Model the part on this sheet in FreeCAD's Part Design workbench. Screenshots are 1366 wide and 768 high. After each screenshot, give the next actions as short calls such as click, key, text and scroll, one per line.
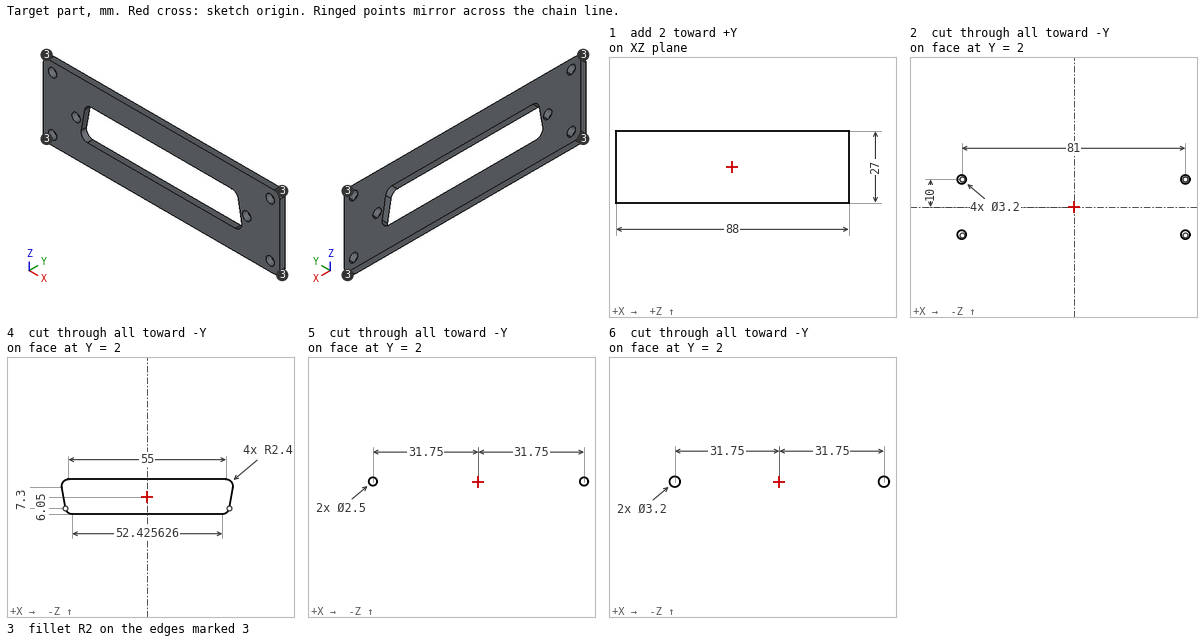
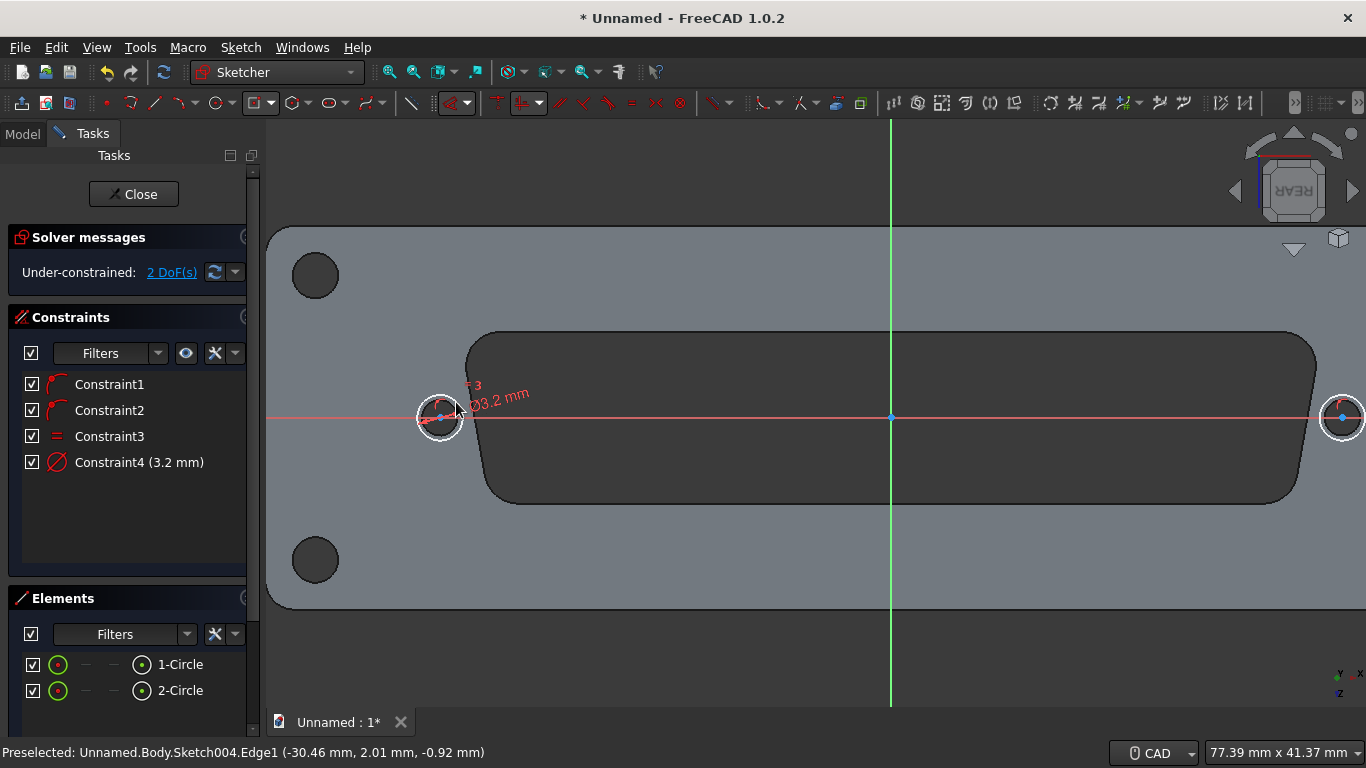
click(440, 418)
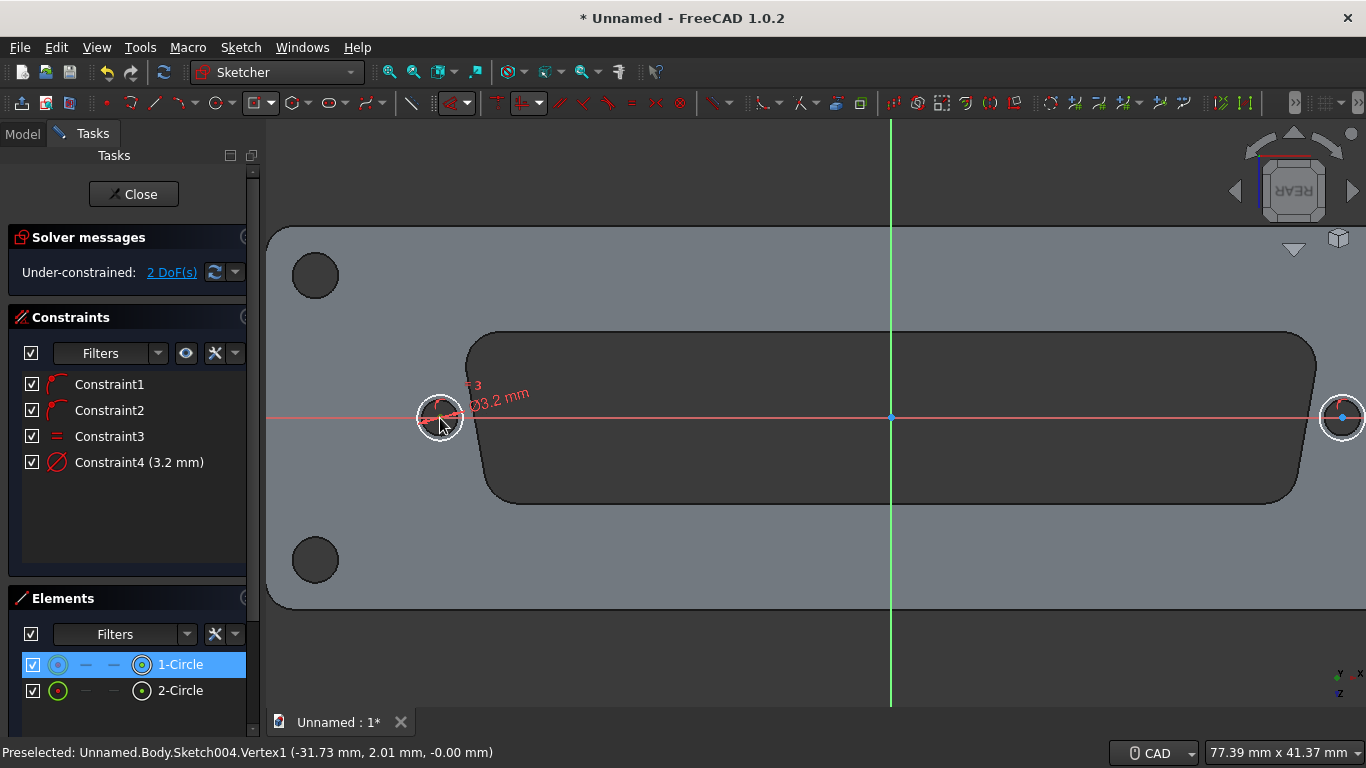
key(l)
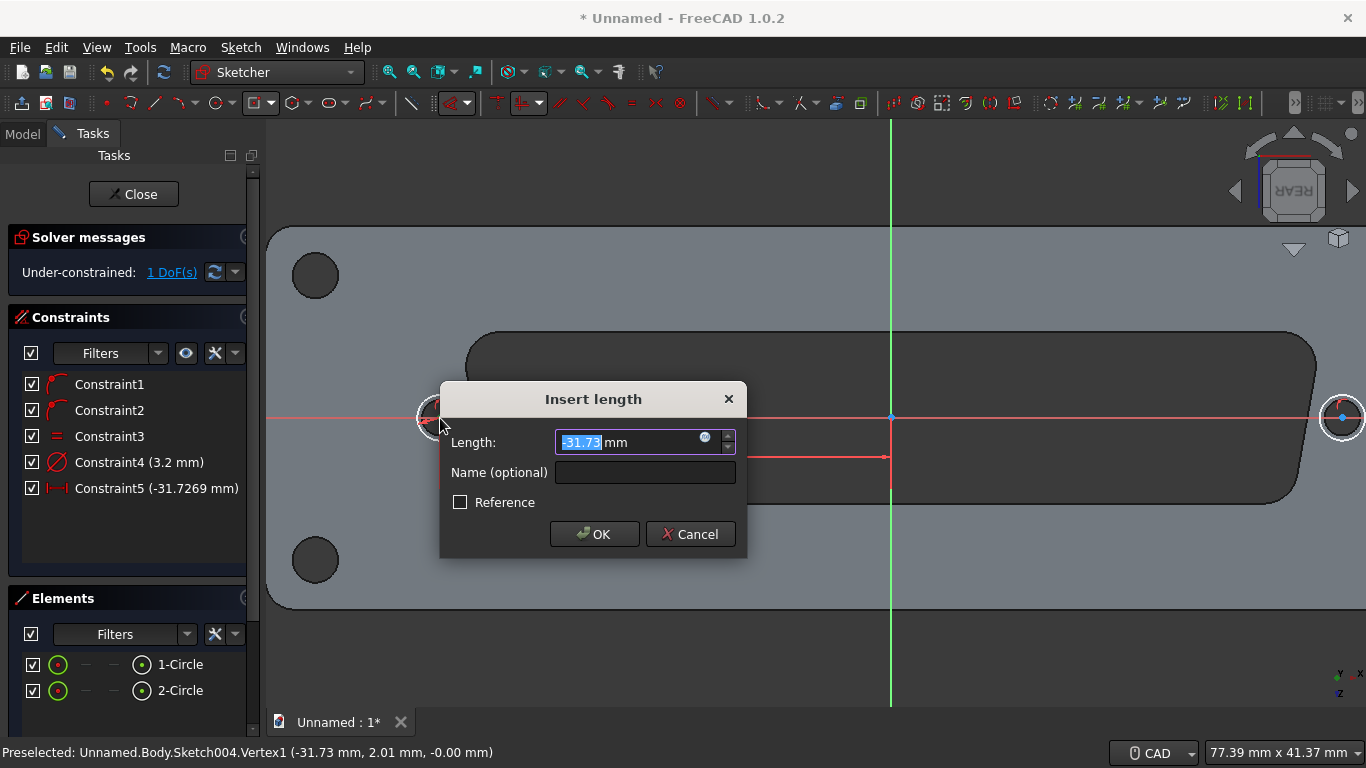
text(-31.75)
key(Return)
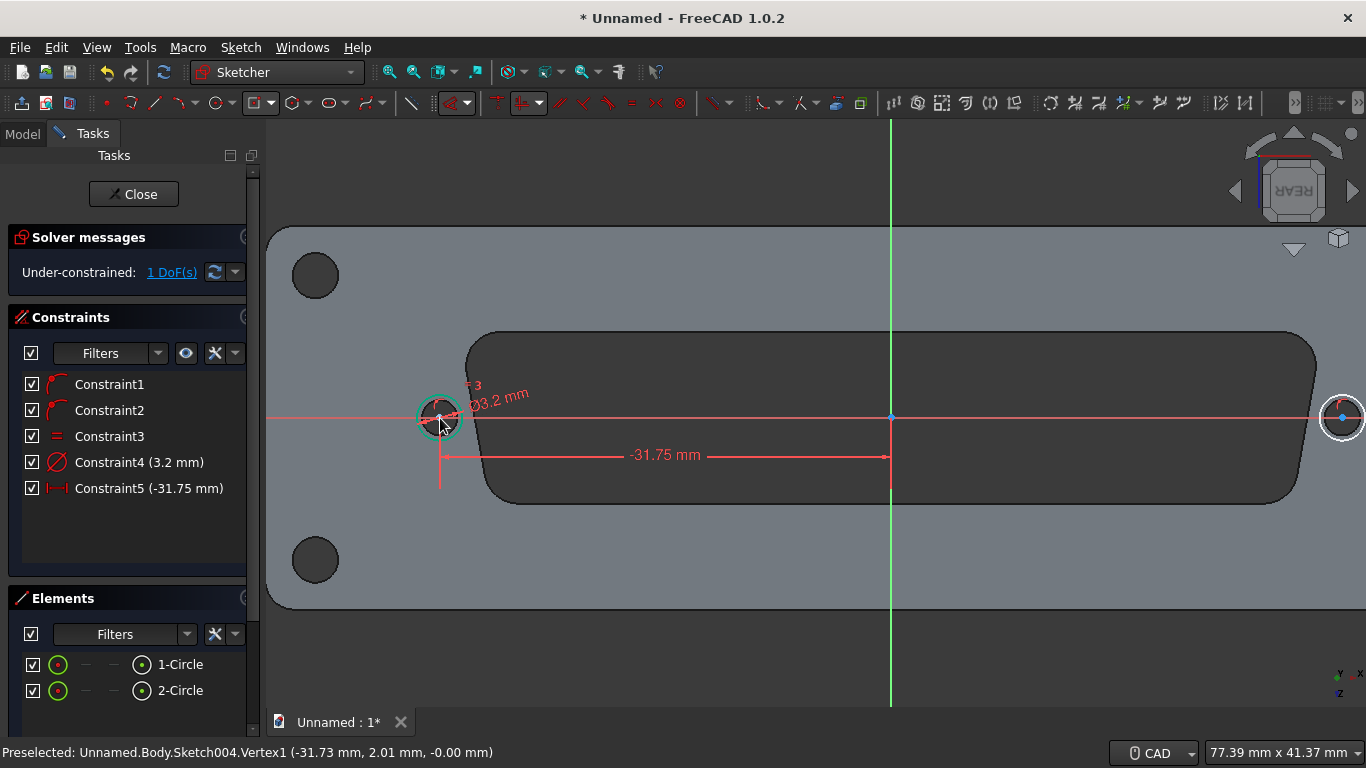
scroll(456, 403, down, 2)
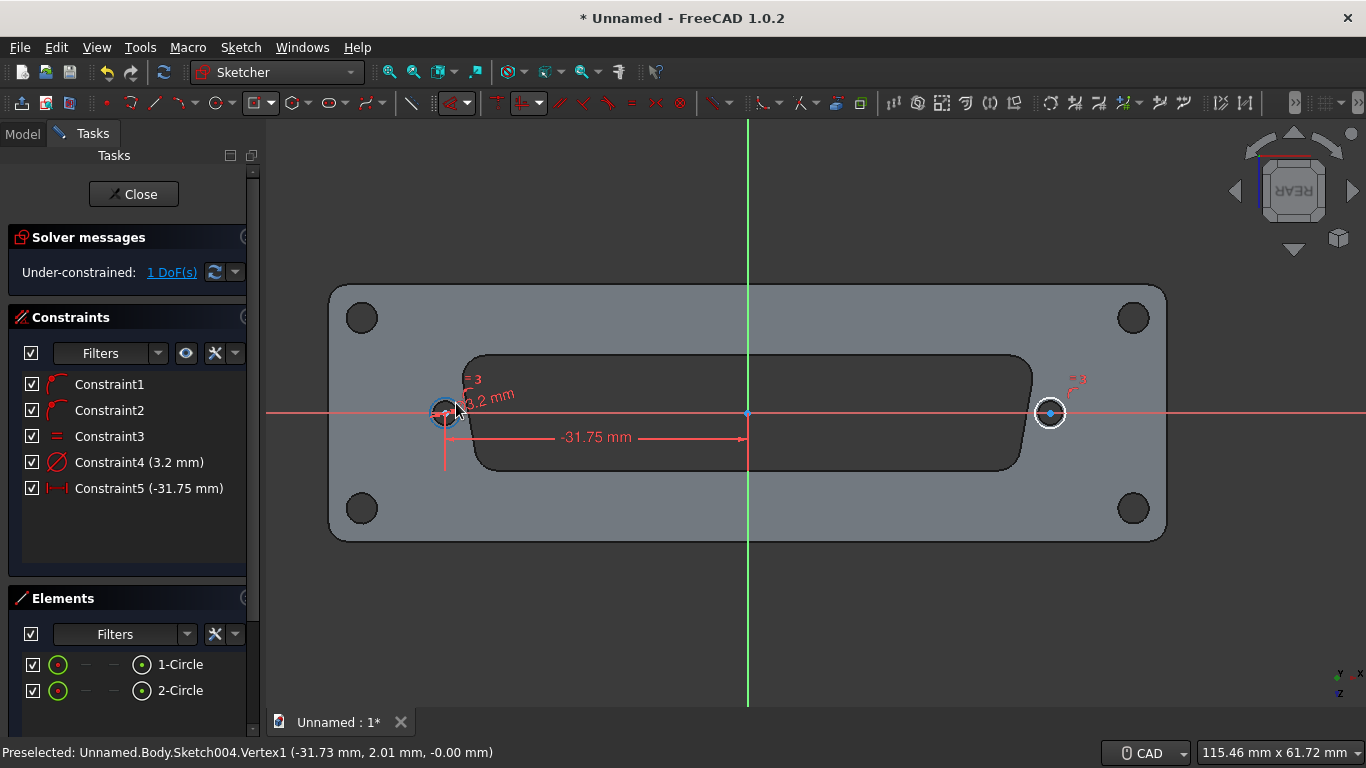
click(1050, 413)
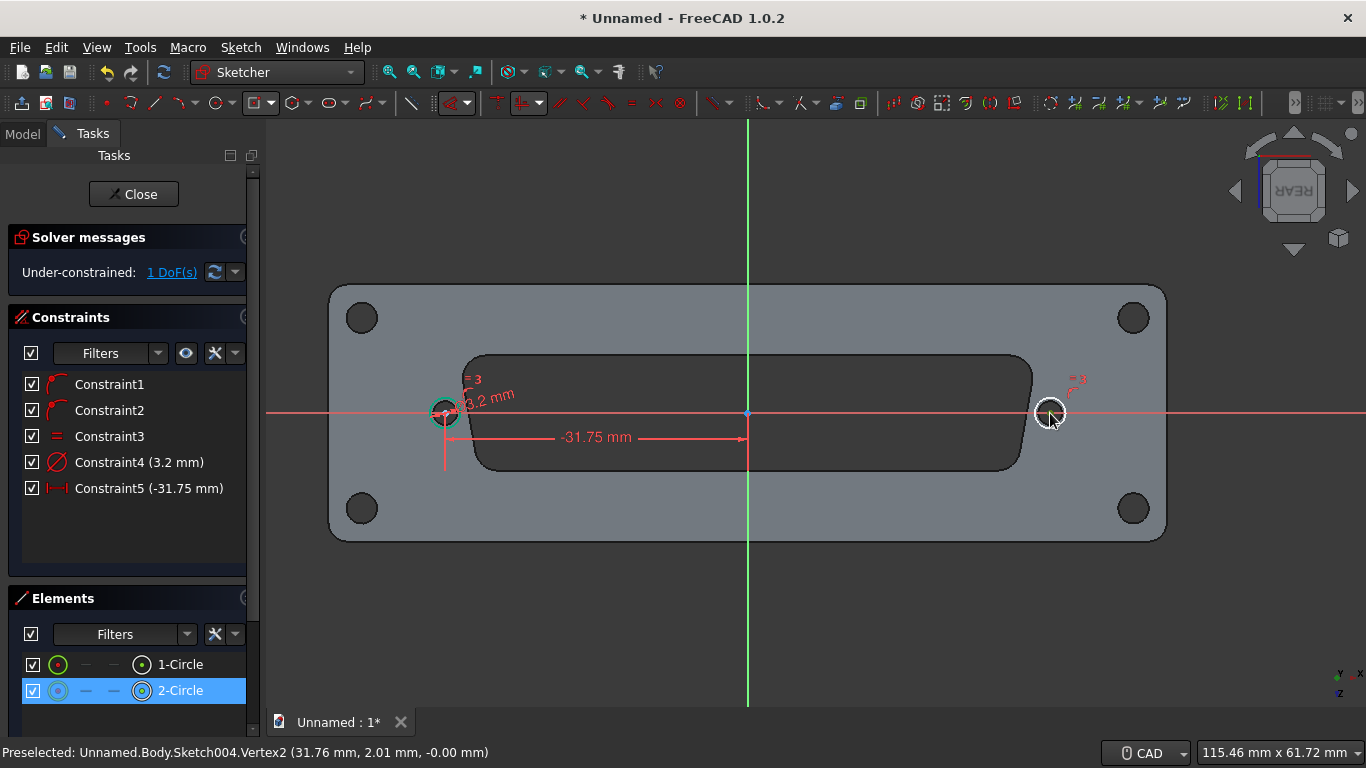
click(470, 104)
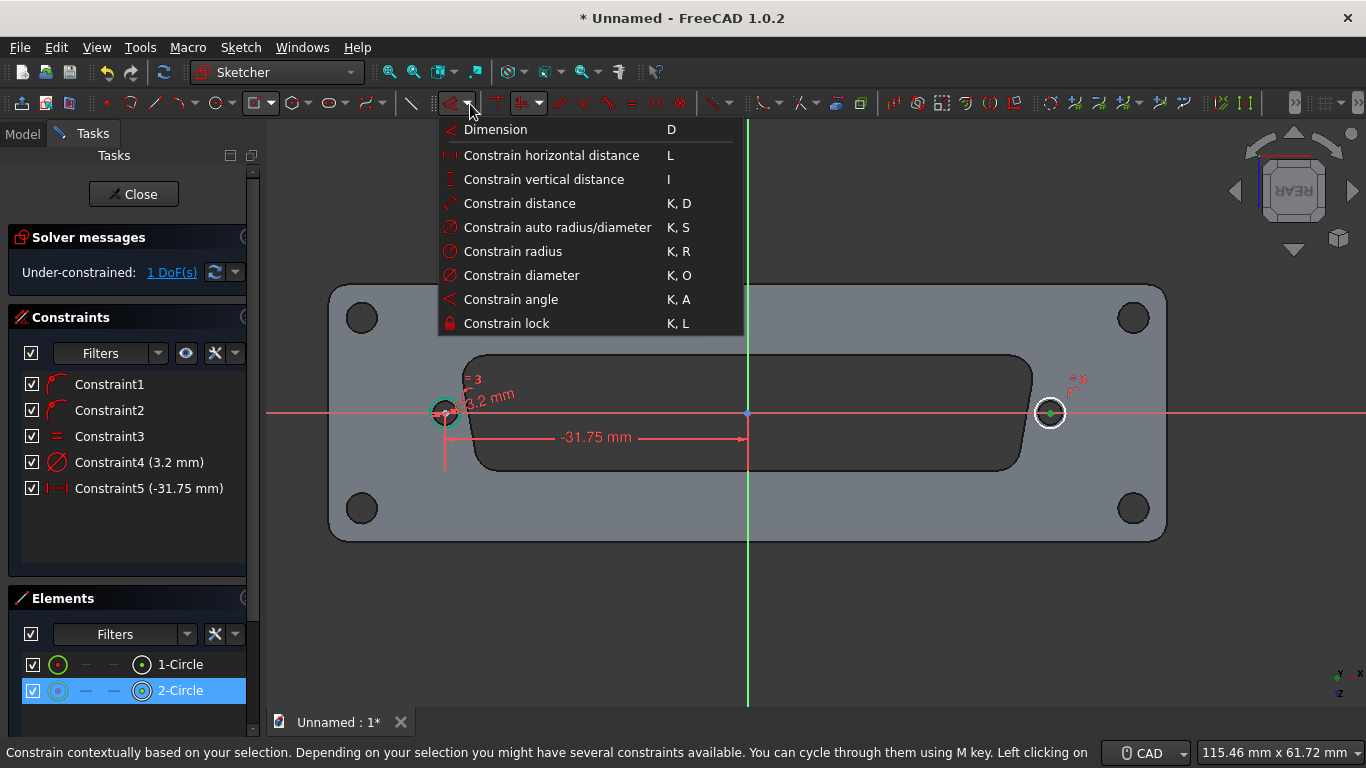
click(591, 155)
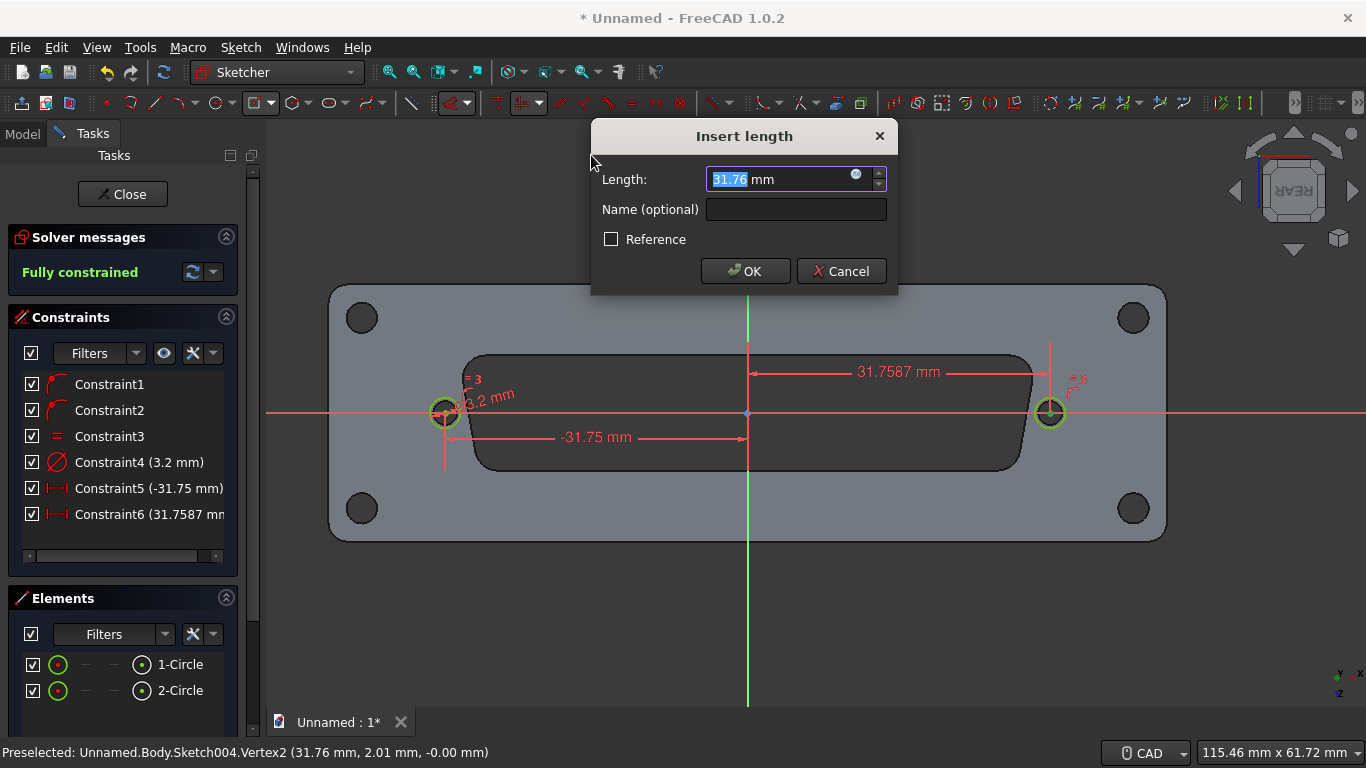
text(31.75)
key(Return)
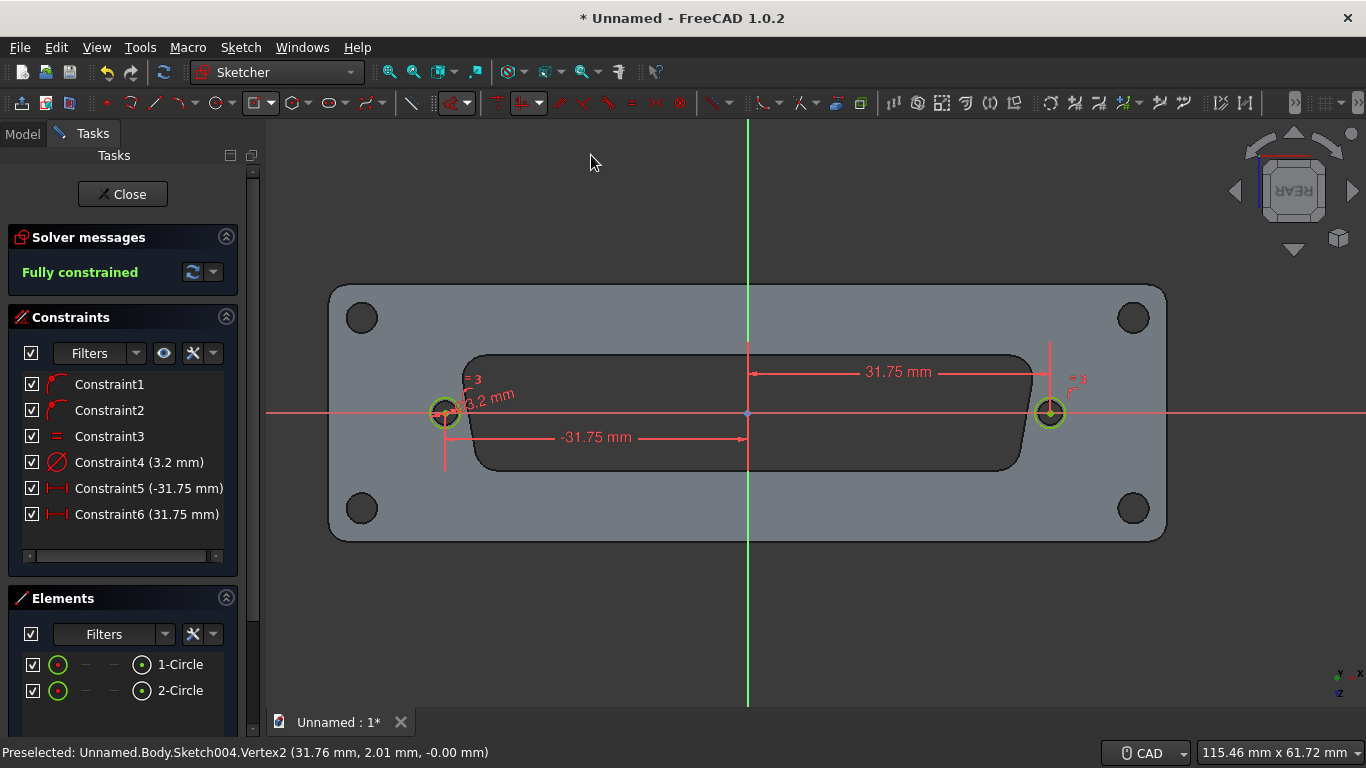
click(123, 194)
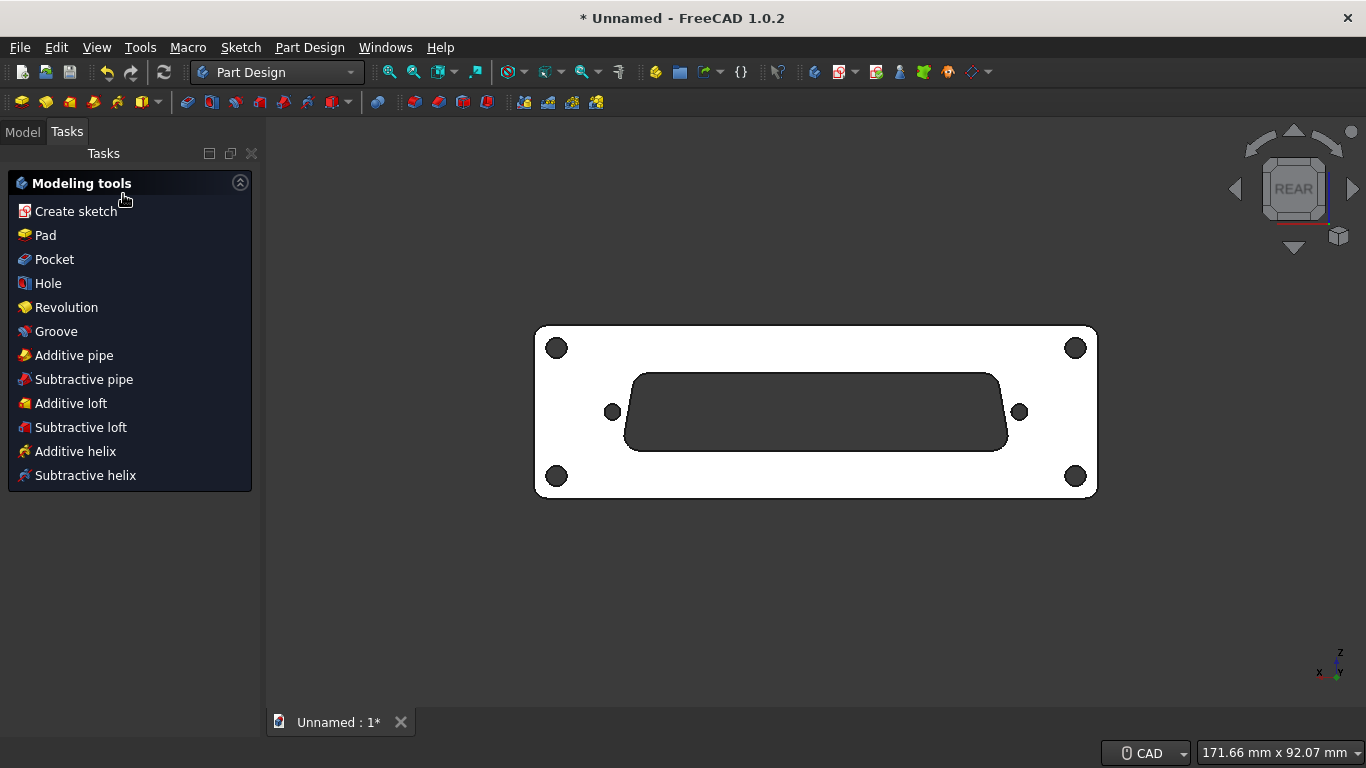
click(188, 102)